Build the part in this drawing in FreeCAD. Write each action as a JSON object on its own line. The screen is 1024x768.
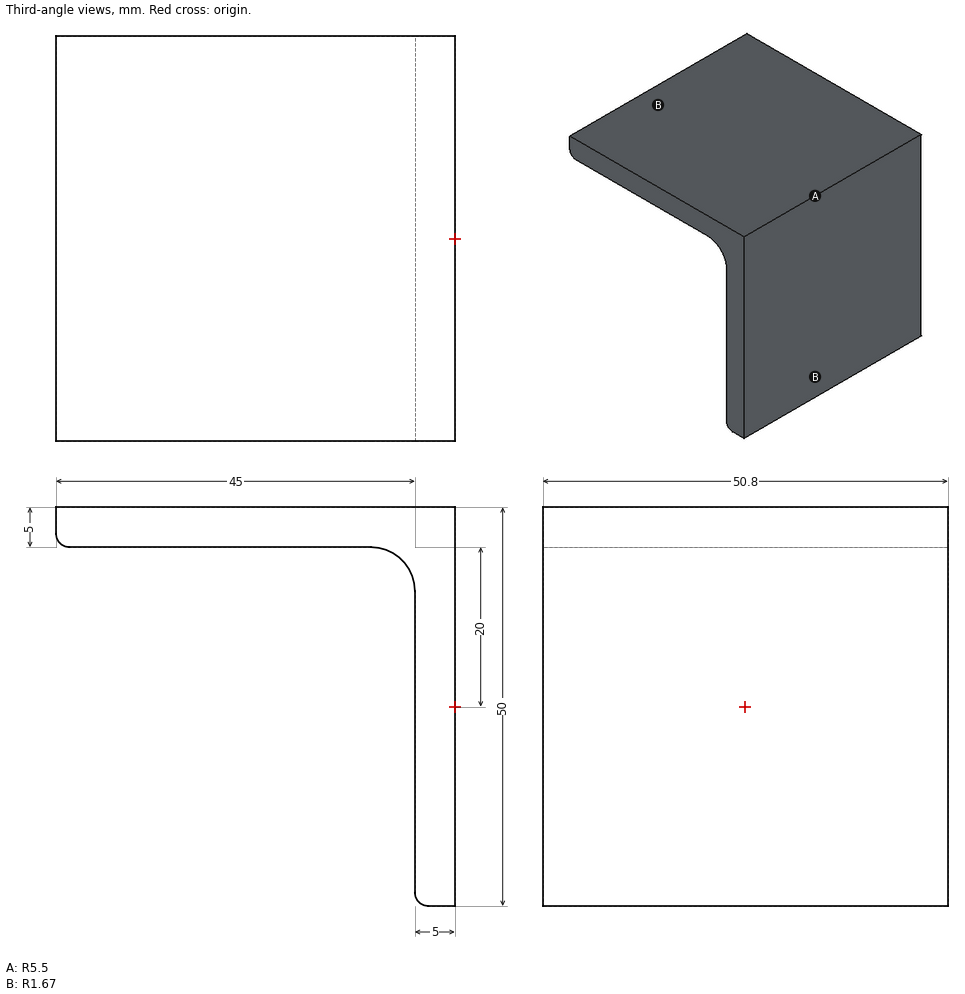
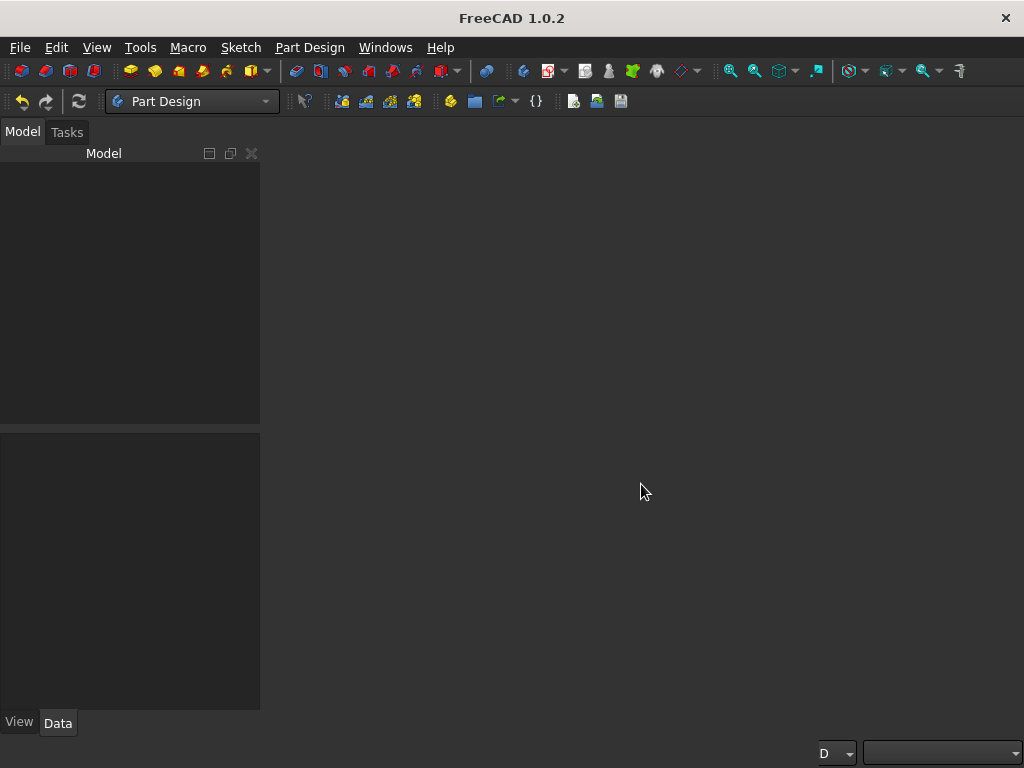
{"action": "left_click", "coordinate": [574, 102]}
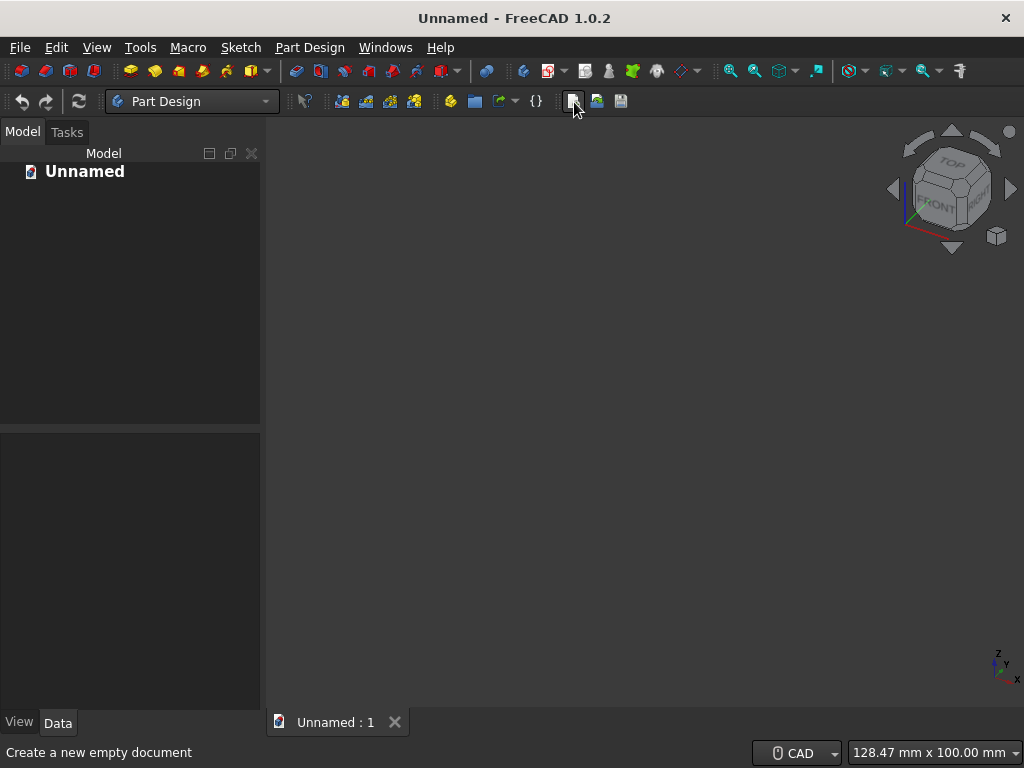
{"action": "left_click", "coordinate": [548, 72]}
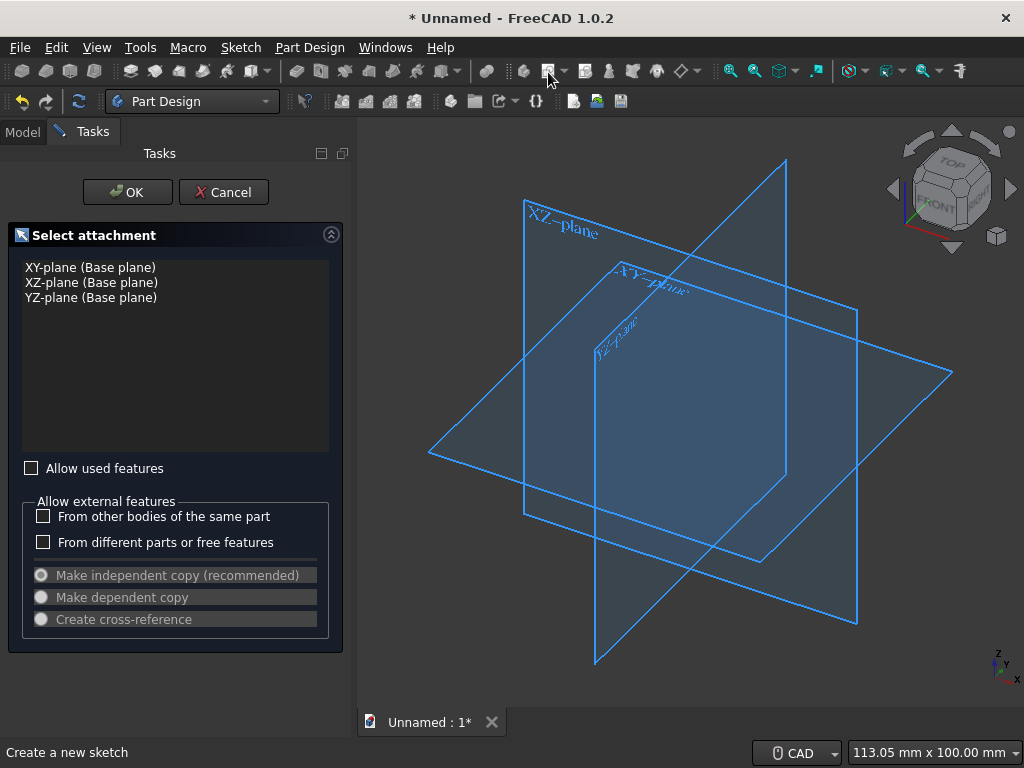
{"action": "left_click", "coordinate": [82, 282]}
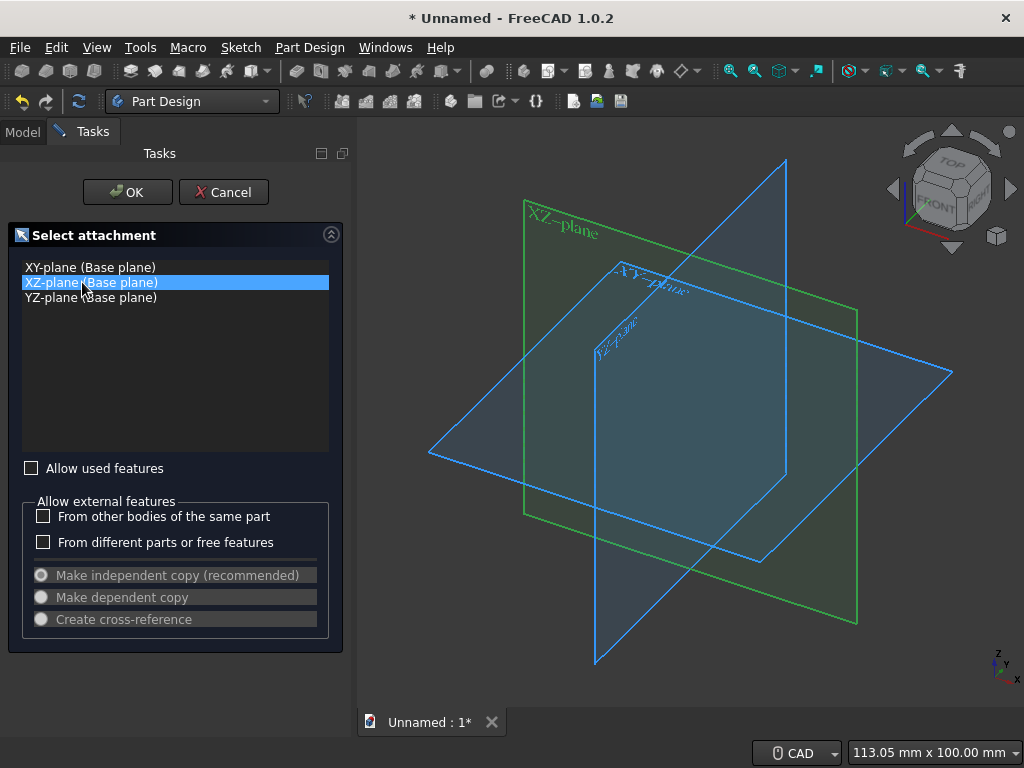
{"action": "left_click", "coordinate": [128, 192]}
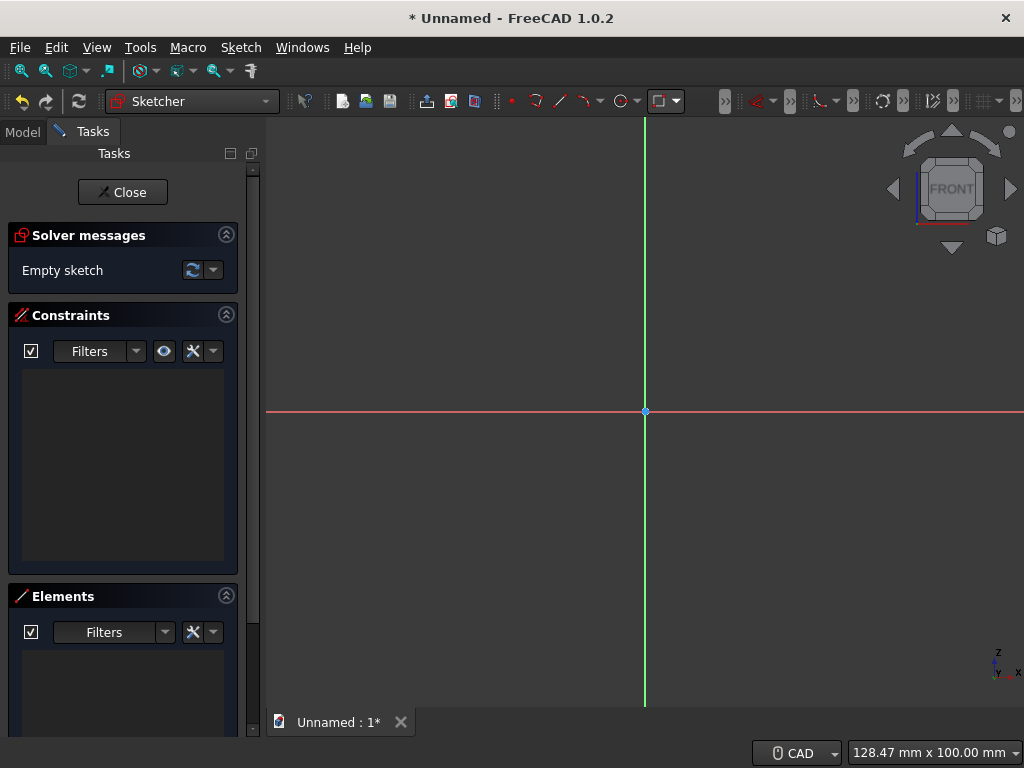
{"action": "left_click", "coordinate": [536, 102]}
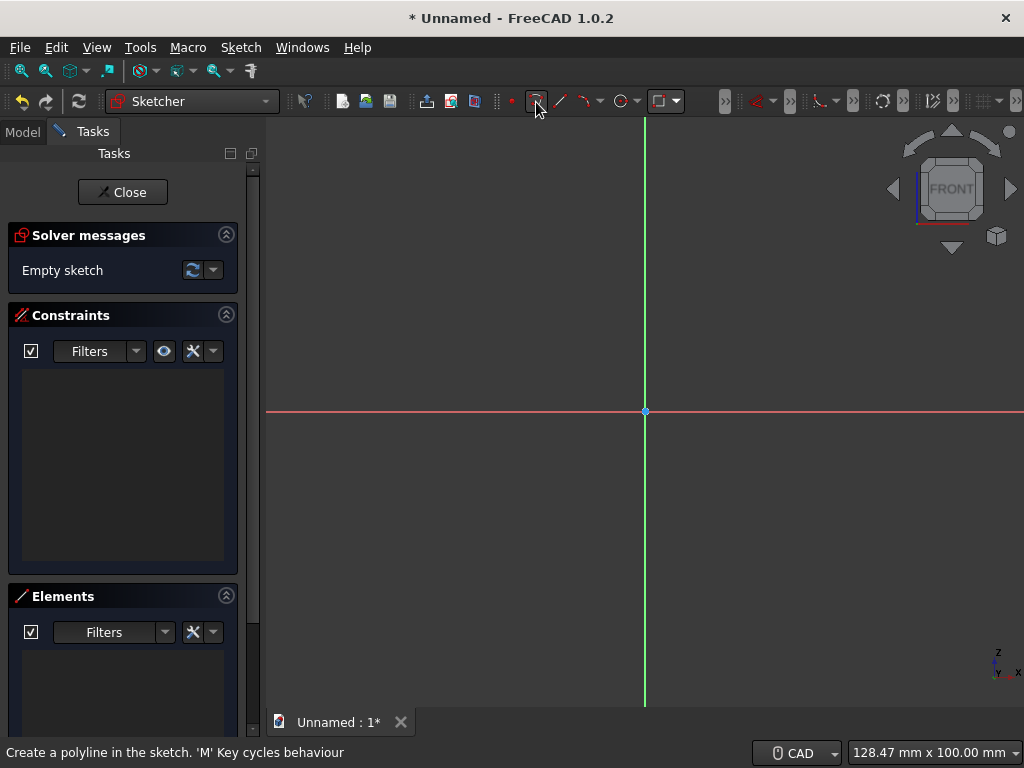
{"action": "left_click", "coordinate": [616, 294]}
{"action": "left_click", "coordinate": [350, 294]}
{"action": "left_click", "coordinate": [350, 264]}
{"action": "left_click", "coordinate": [645, 264]}
{"action": "left_click", "coordinate": [636, 560]}
{"action": "left_click", "coordinate": [616, 560]}
{"action": "left_click", "coordinate": [616, 295]}
{"action": "key", "text": "Escape"}
{"action": "key", "text": "Escape"}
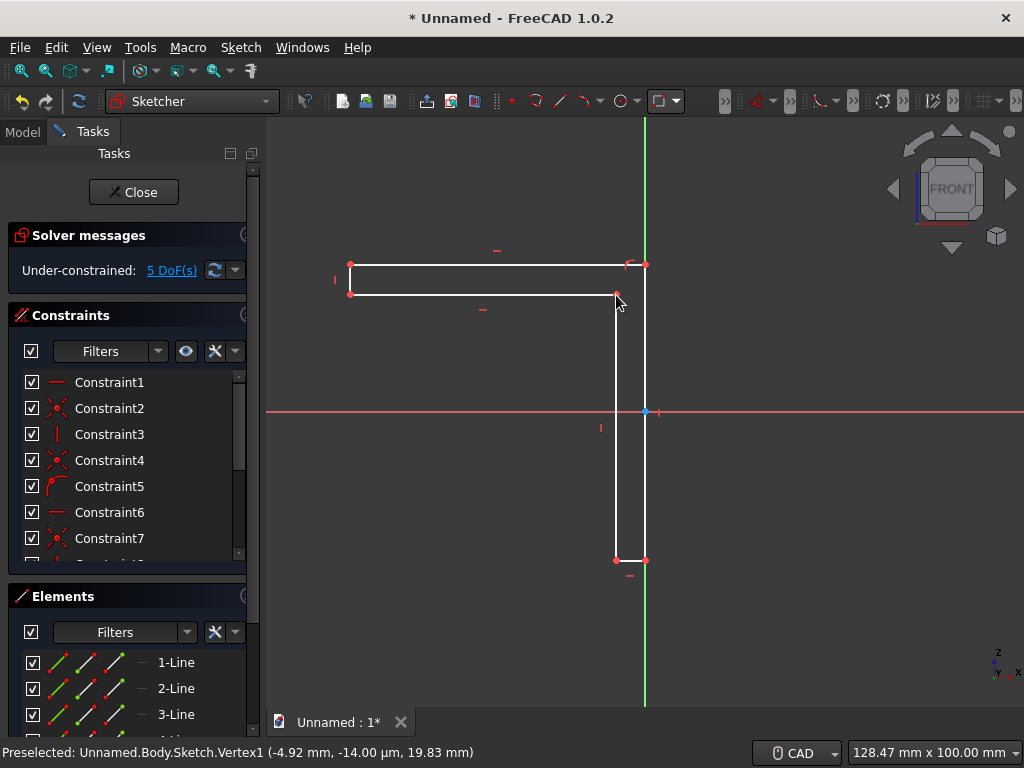
{"action": "left_click", "coordinate": [756, 102]}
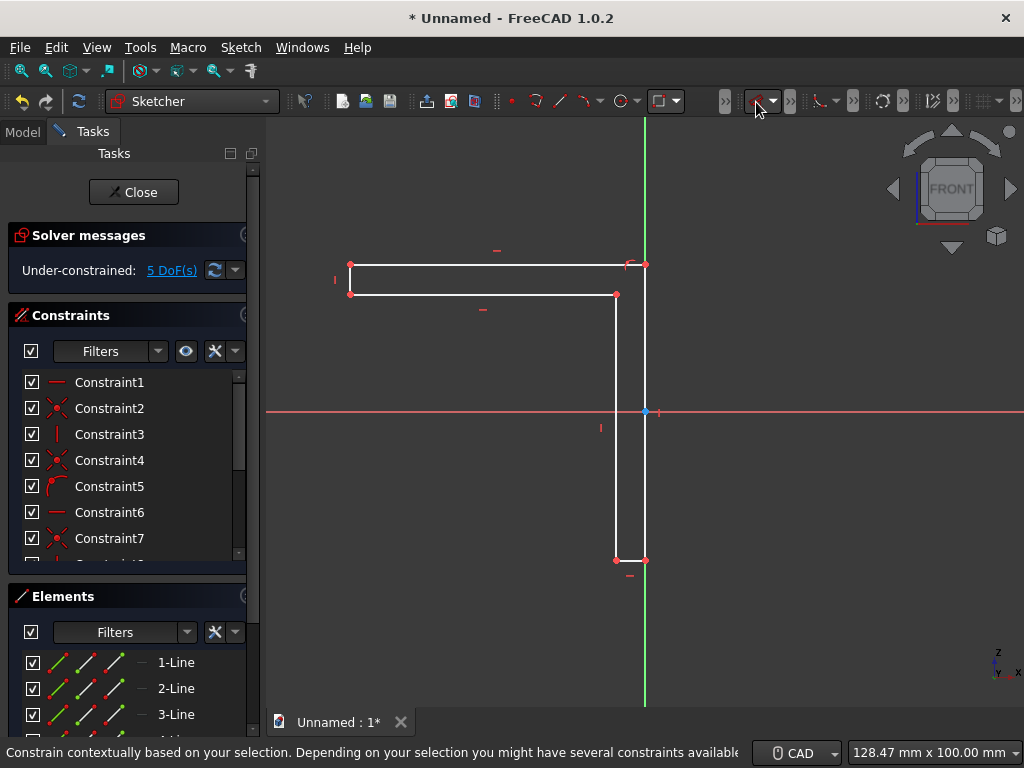
{"action": "scroll", "coordinate": [350, 286], "scroll_direction": "up", "scroll_amount": 3}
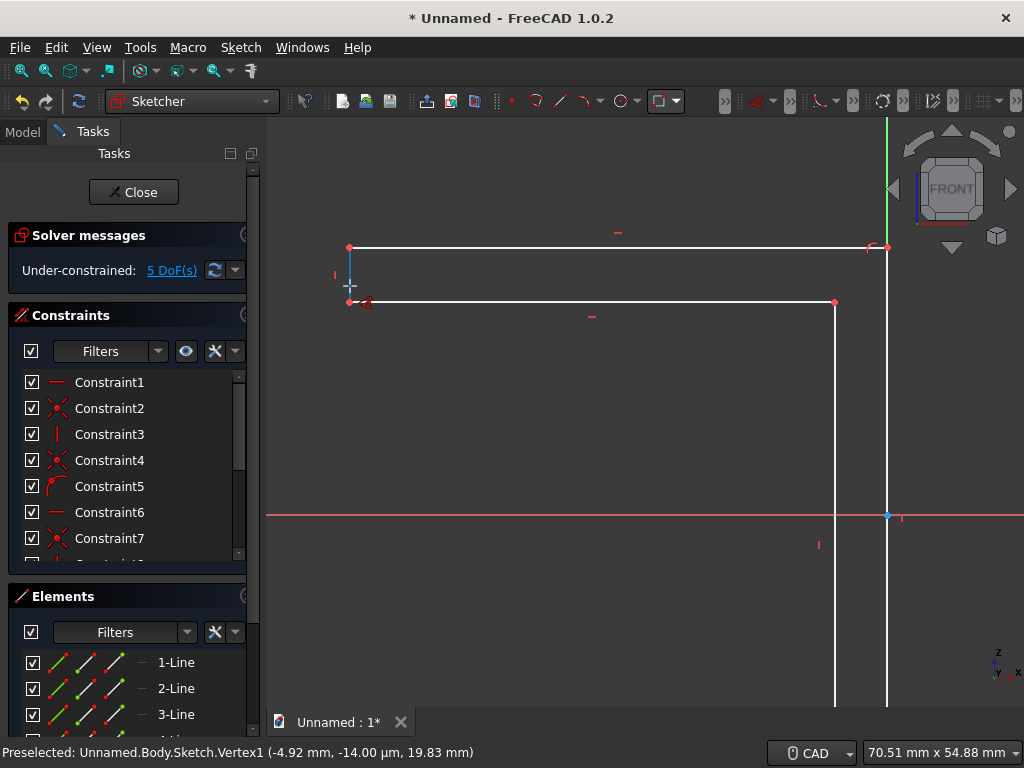
{"action": "left_click", "coordinate": [350, 286]}
{"action": "left_click", "coordinate": [316, 275]}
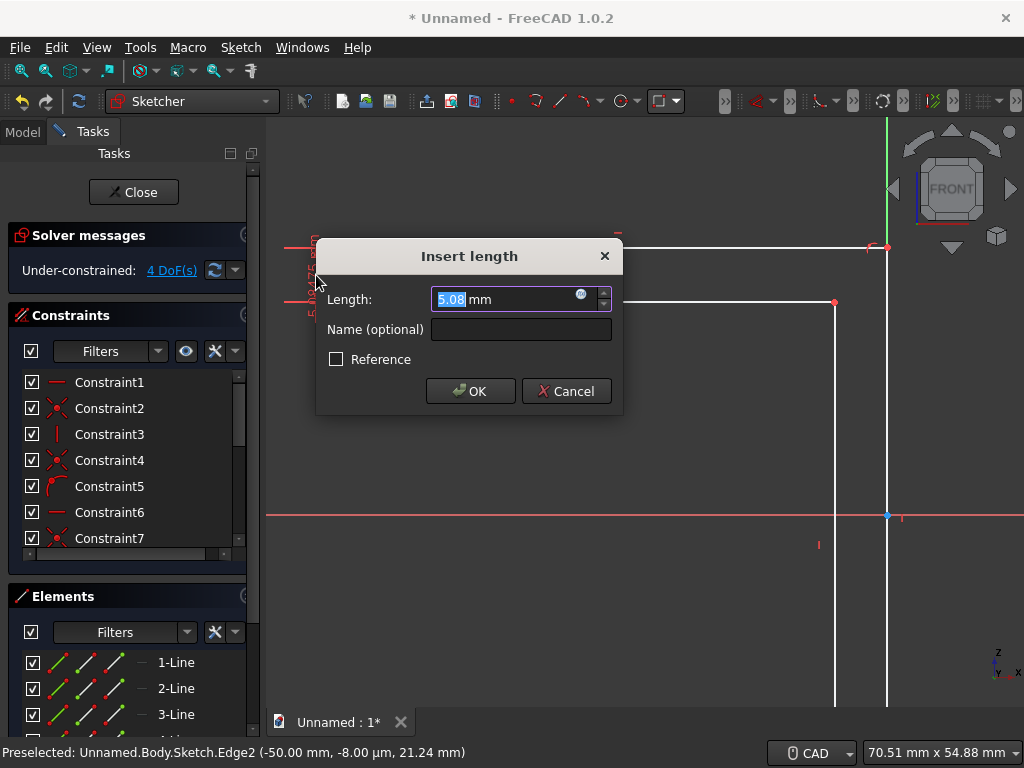
{"action": "type", "text": "5"}
{"action": "key", "text": "Return"}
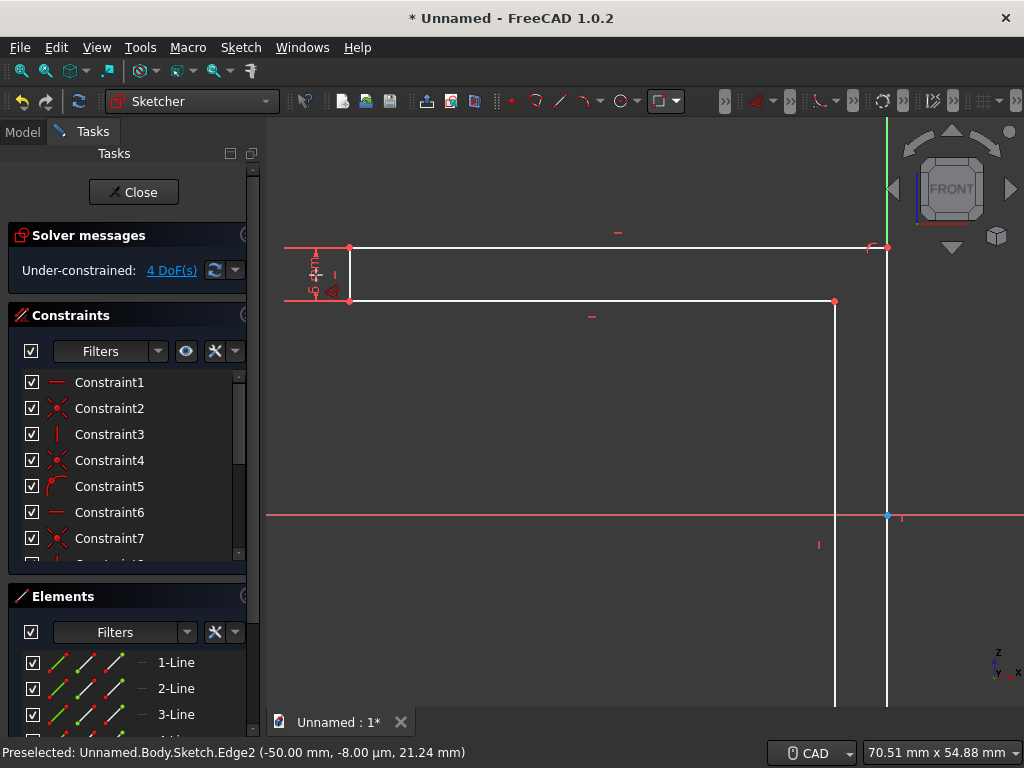
{"action": "scroll", "coordinate": [491, 202], "scroll_direction": "down", "scroll_amount": 2}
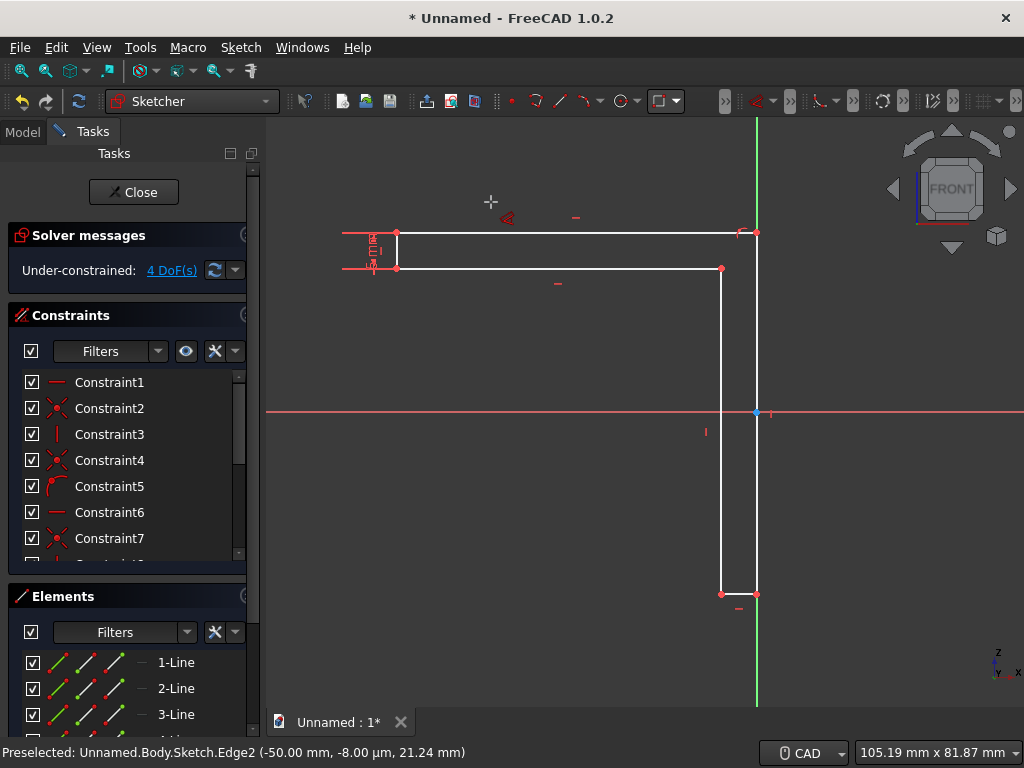
{"action": "scroll", "coordinate": [746, 594], "scroll_direction": "up", "scroll_amount": 2}